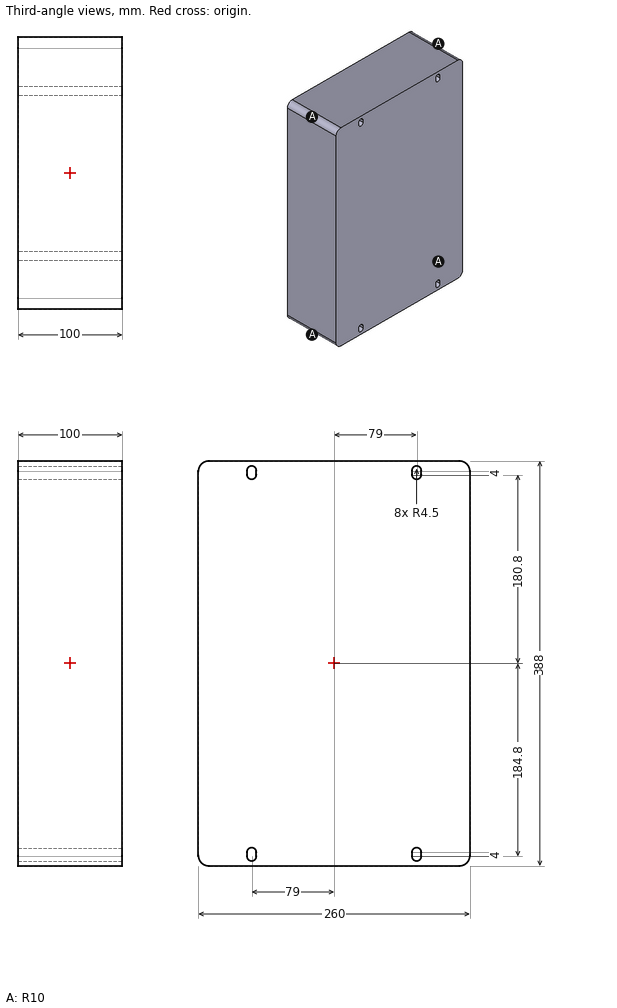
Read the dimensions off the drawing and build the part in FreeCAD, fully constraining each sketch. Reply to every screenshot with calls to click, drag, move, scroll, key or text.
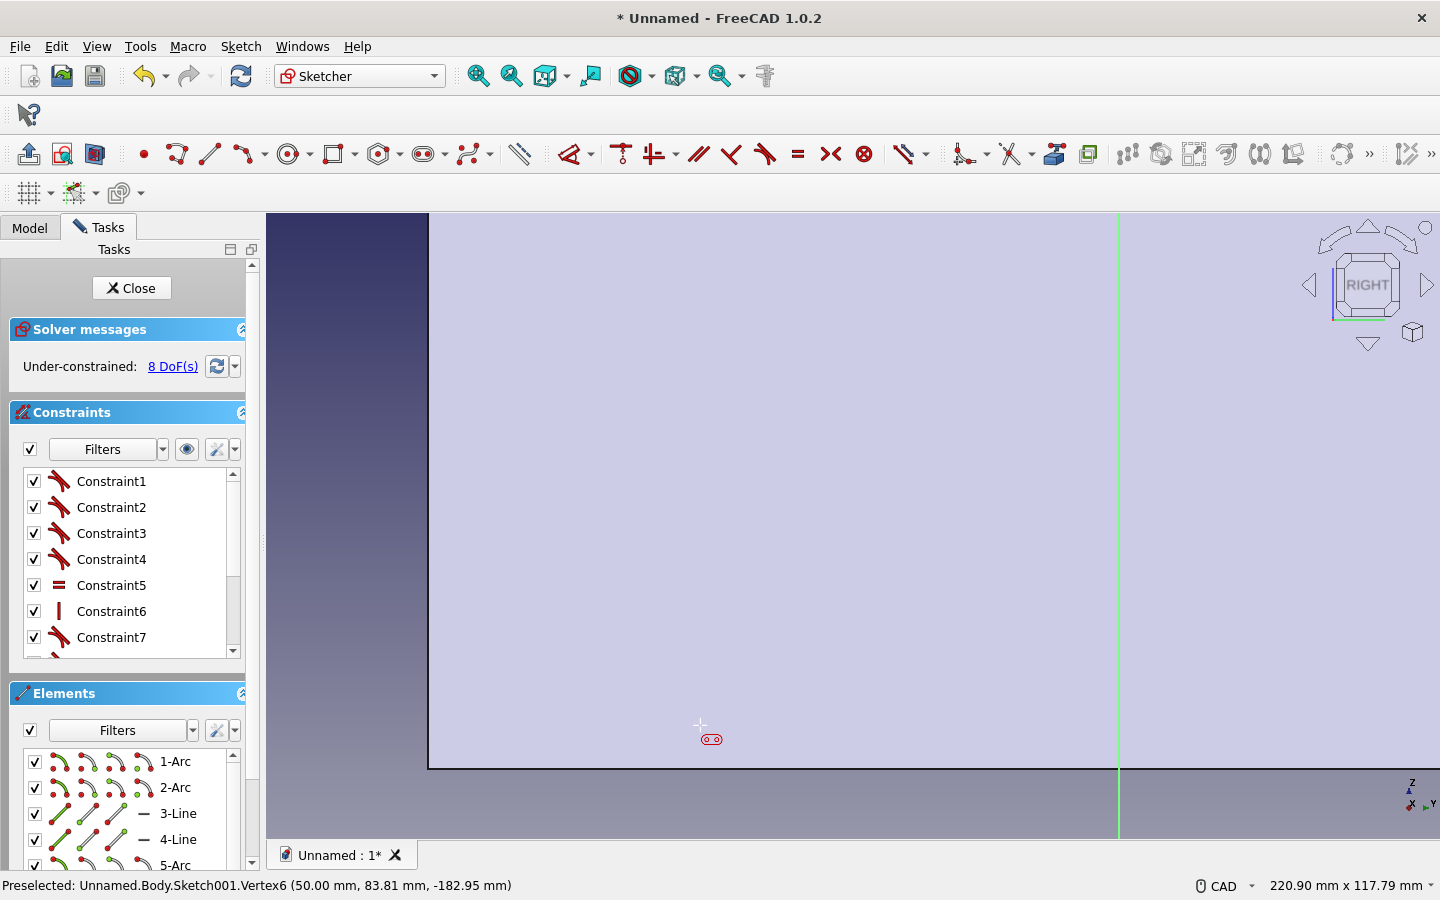
scroll(700, 725, down, 8)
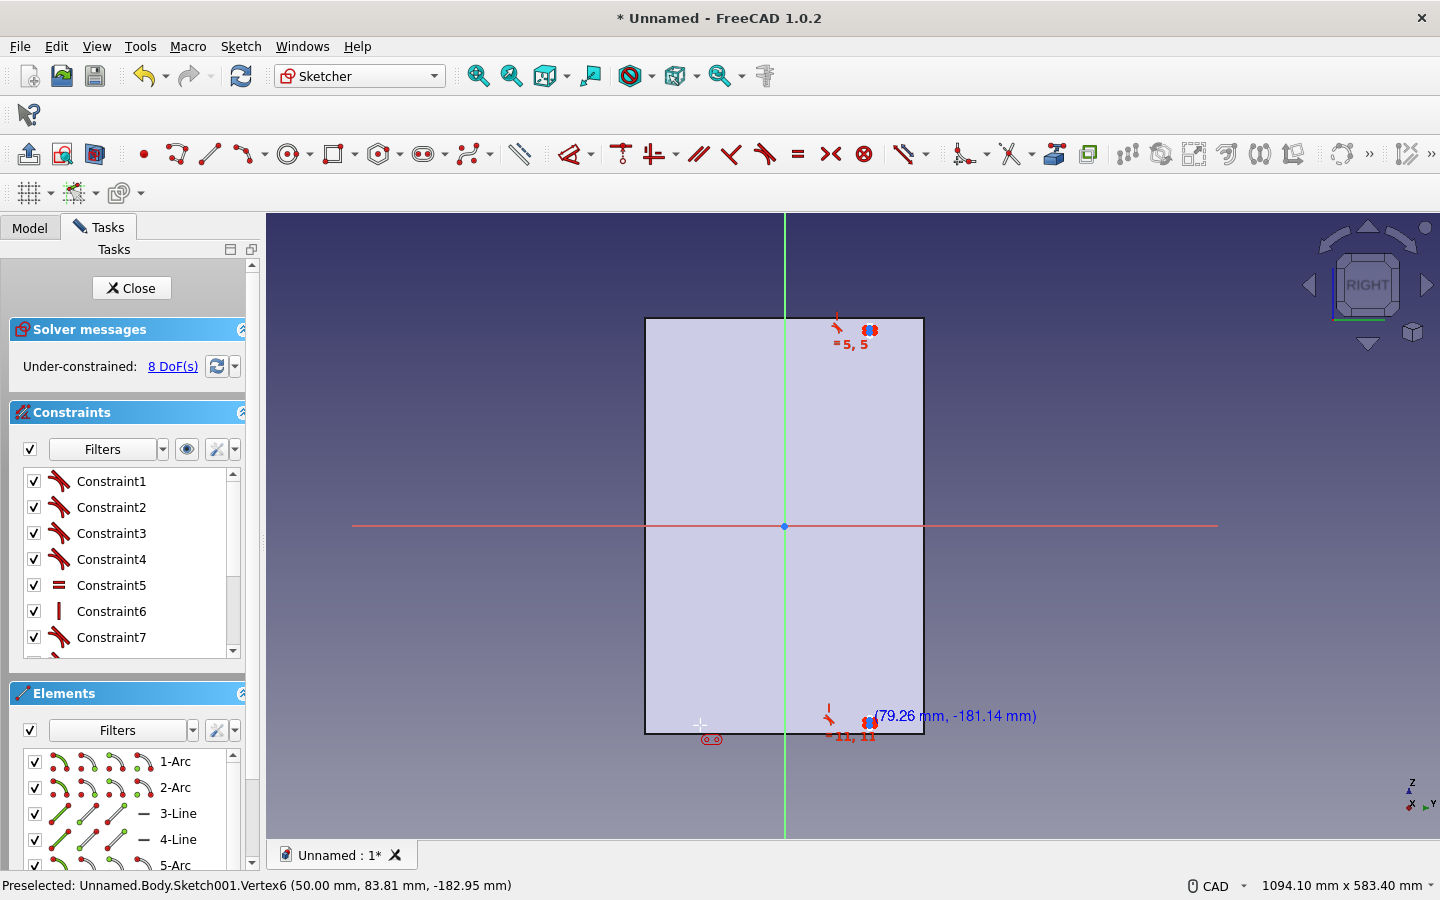
click(700, 725)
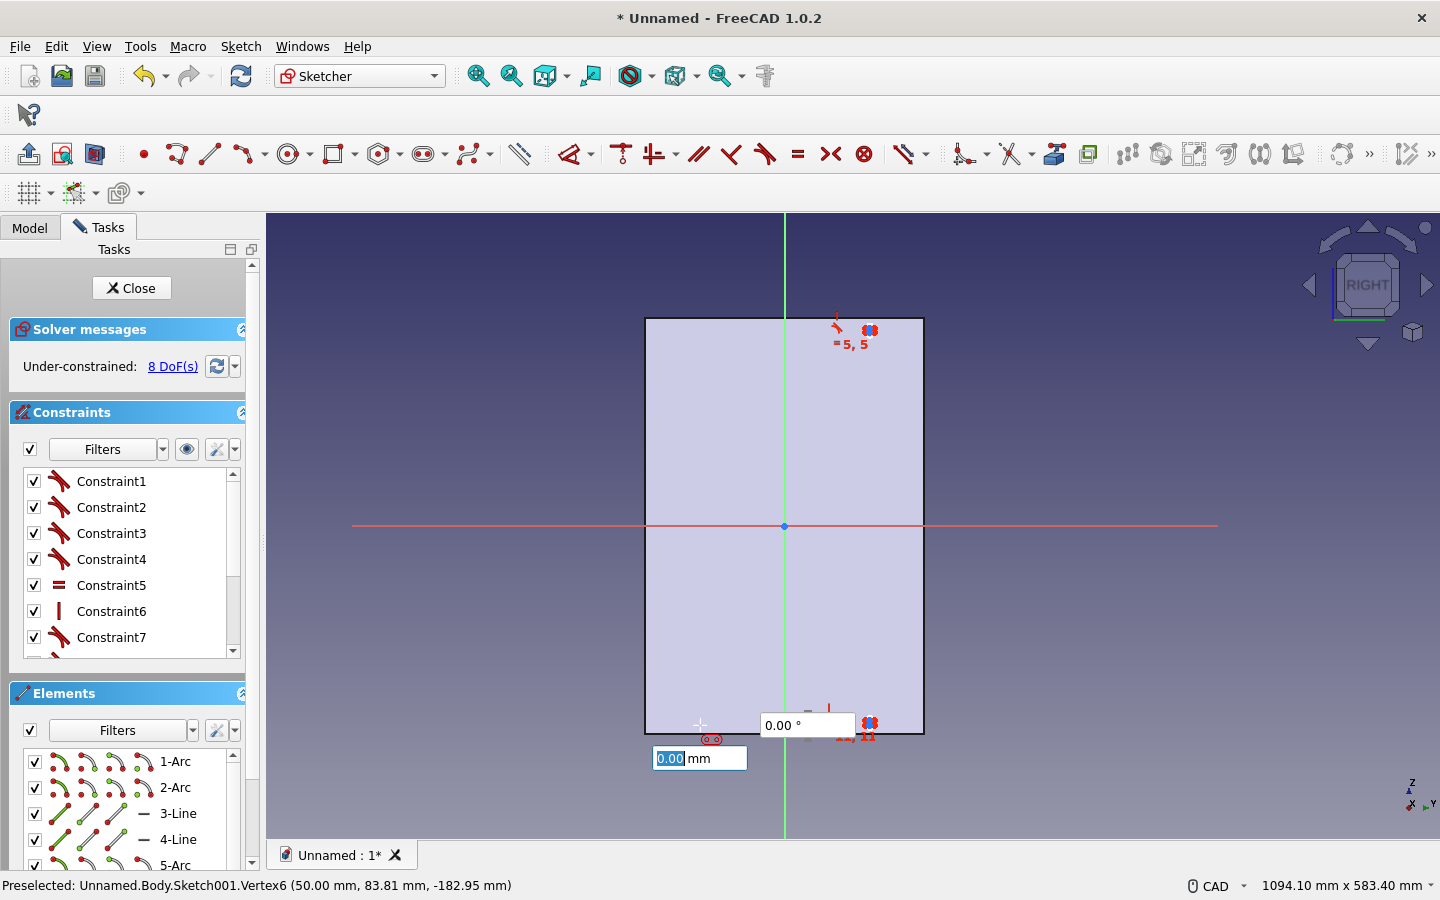
scroll(700, 720, up, 7)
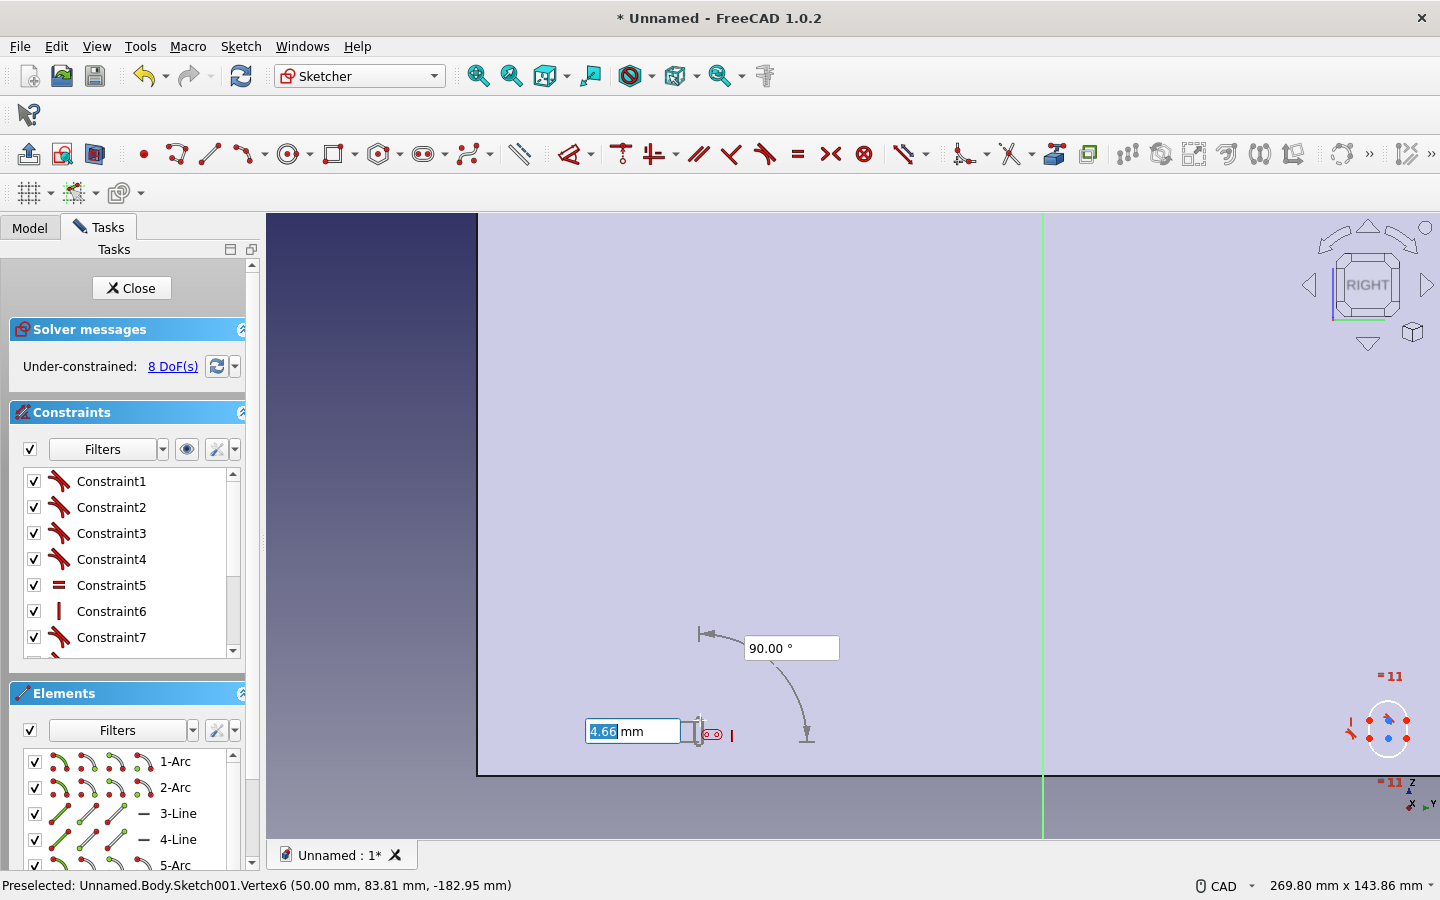
click(699, 719)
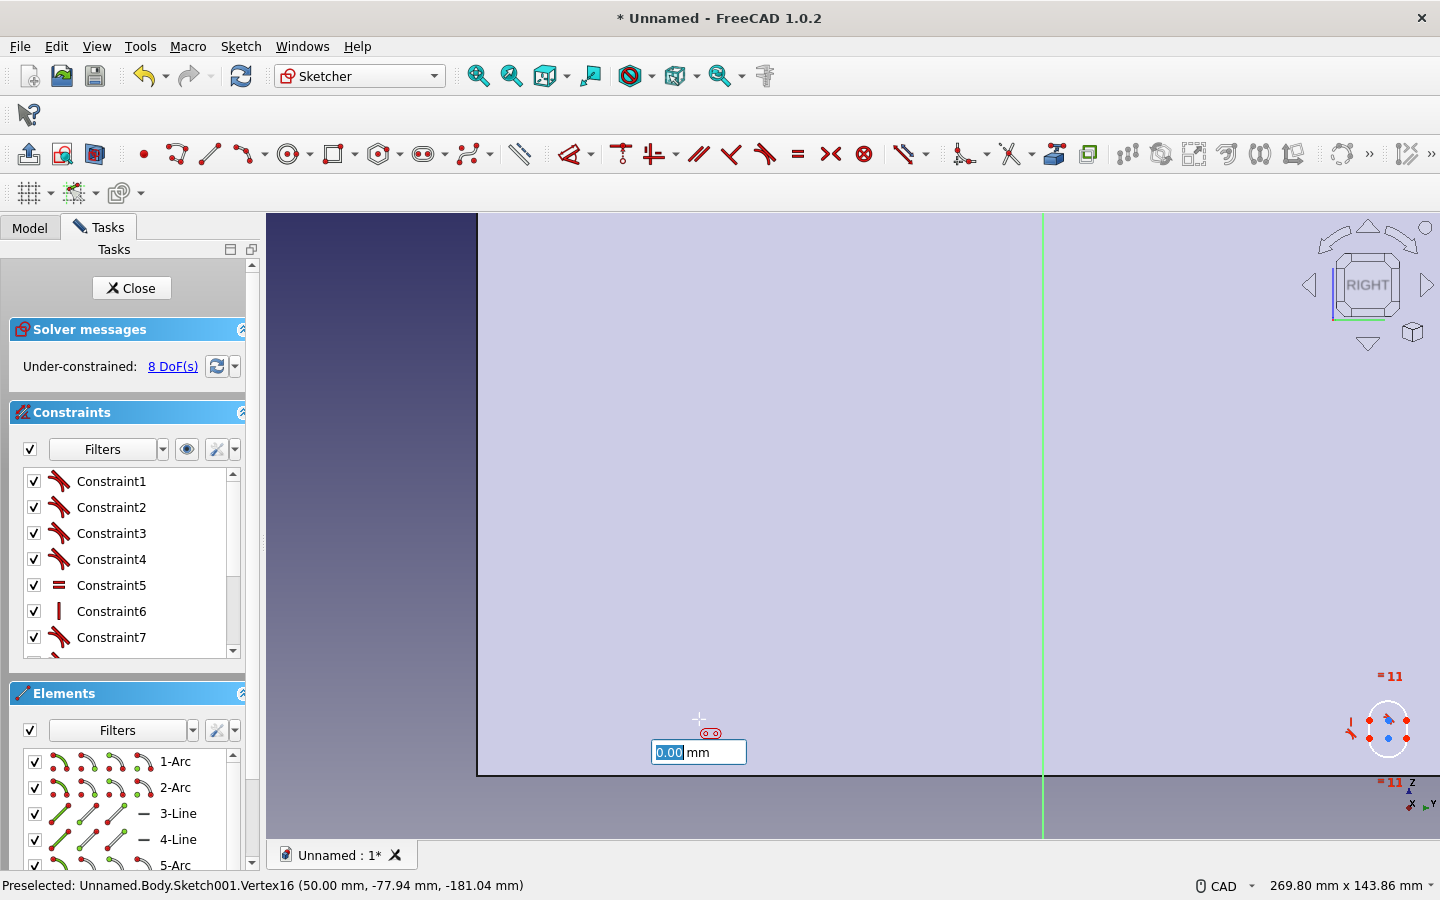
click(719, 727)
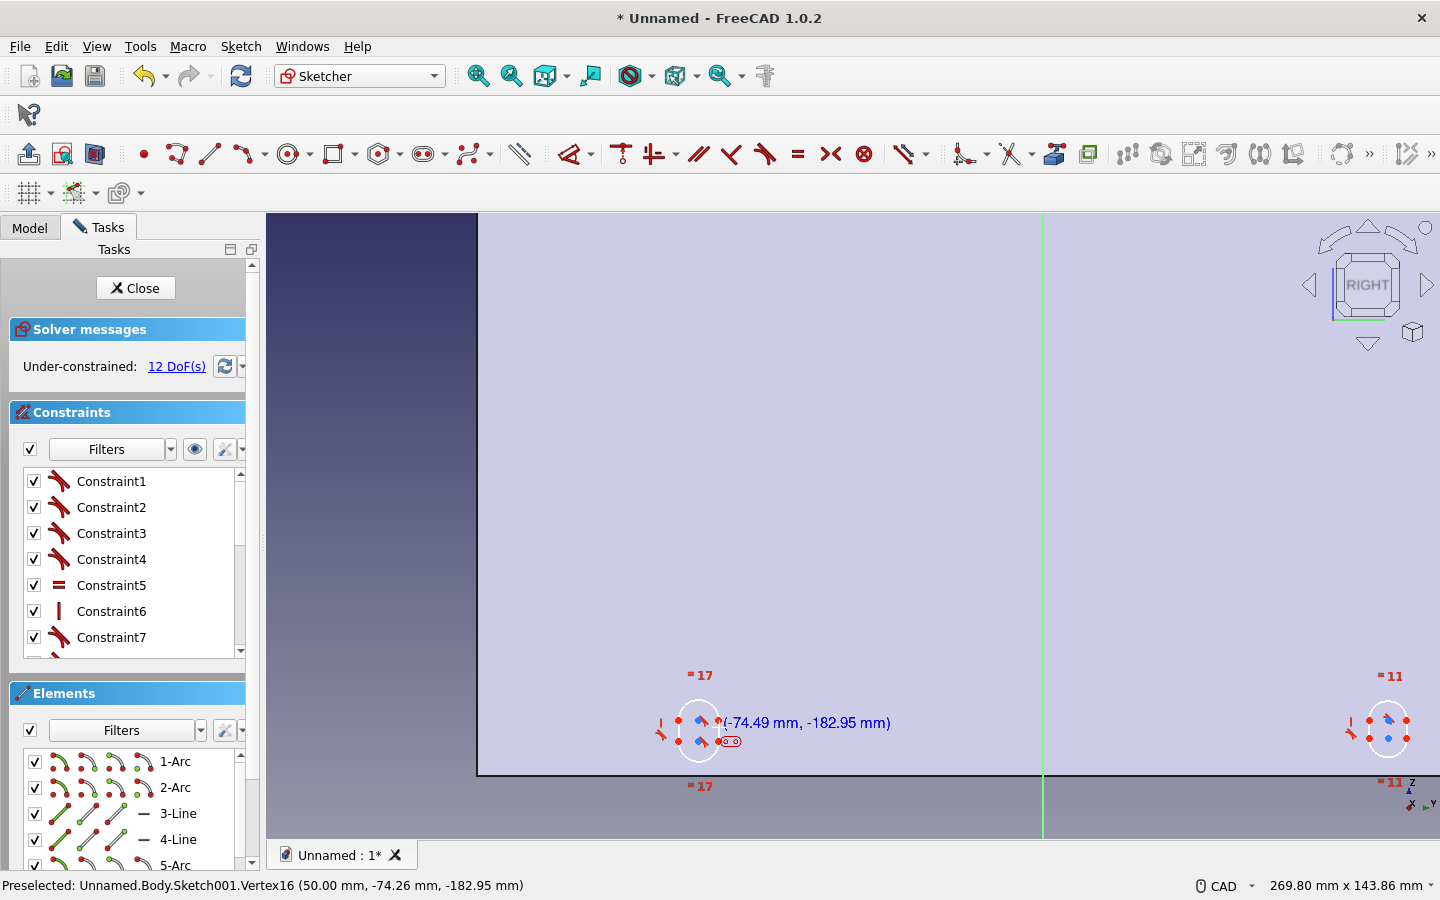
scroll(700, 720, down, 7)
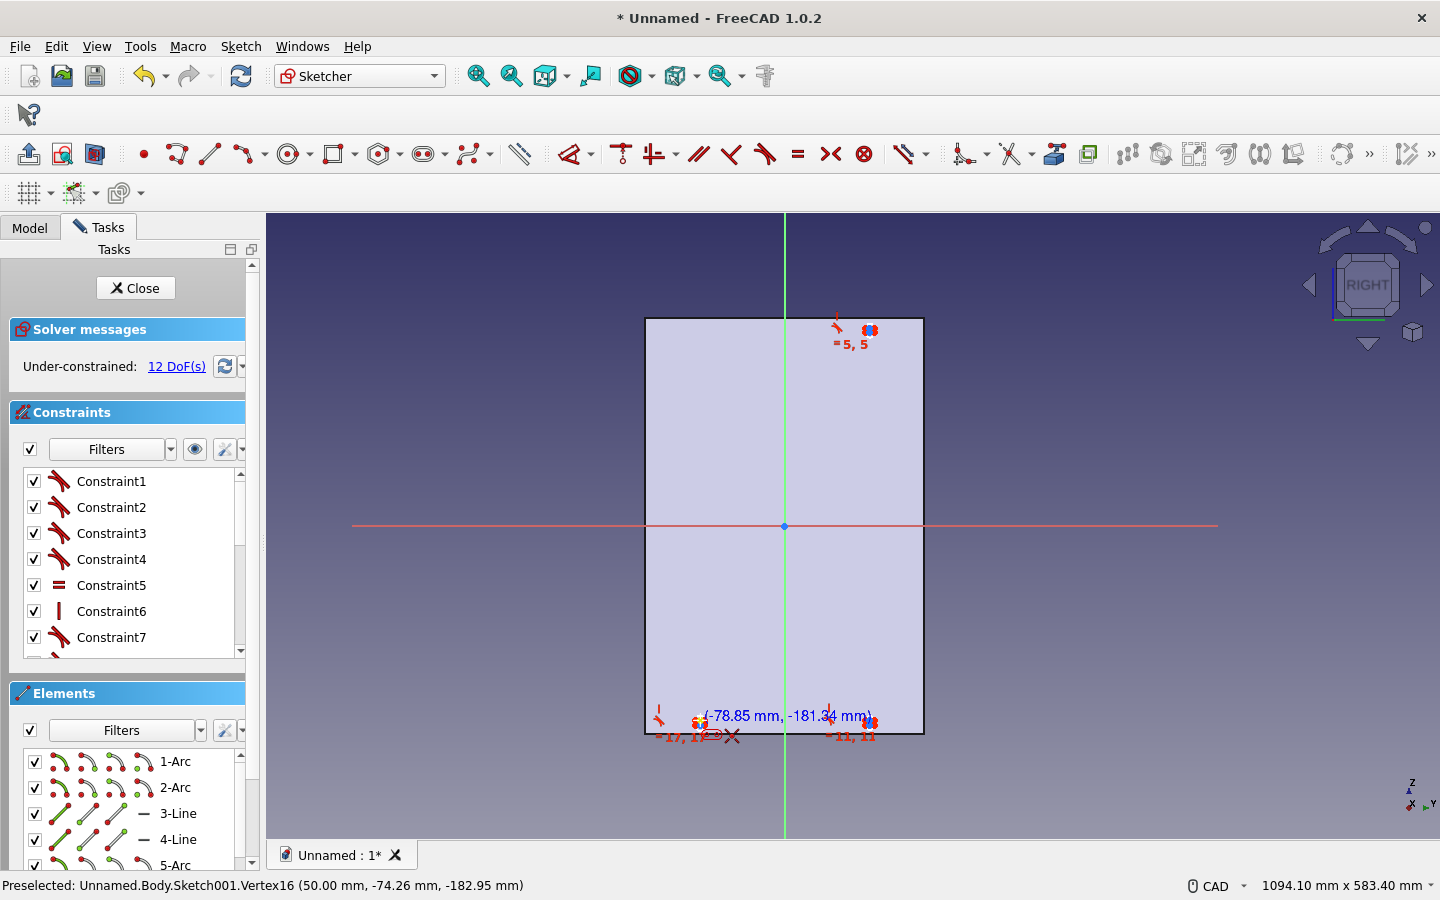
scroll(700, 332, up, 8)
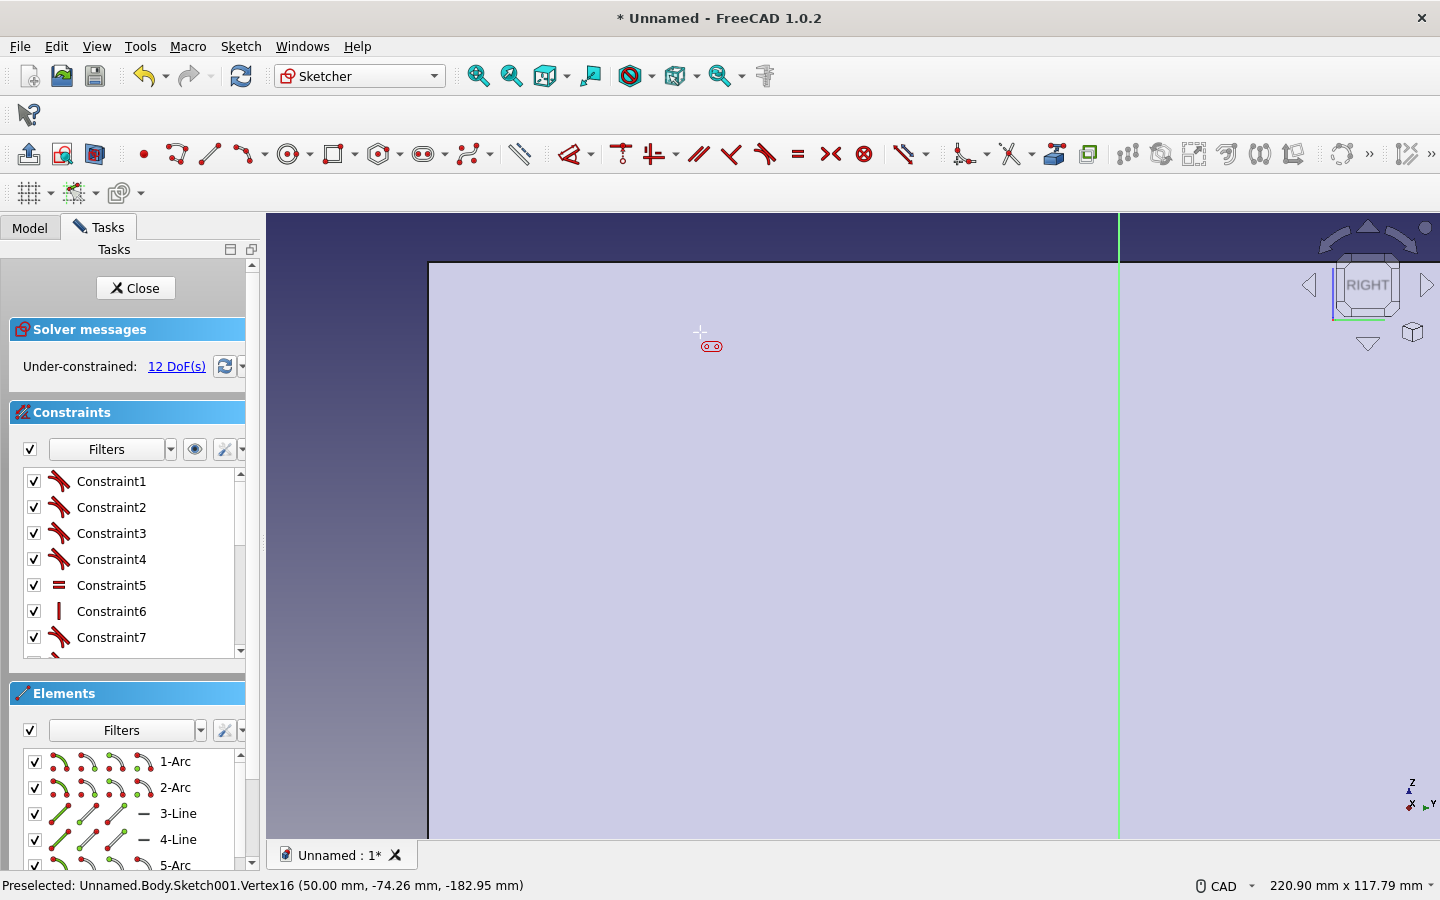
scroll(700, 332, down, 8)